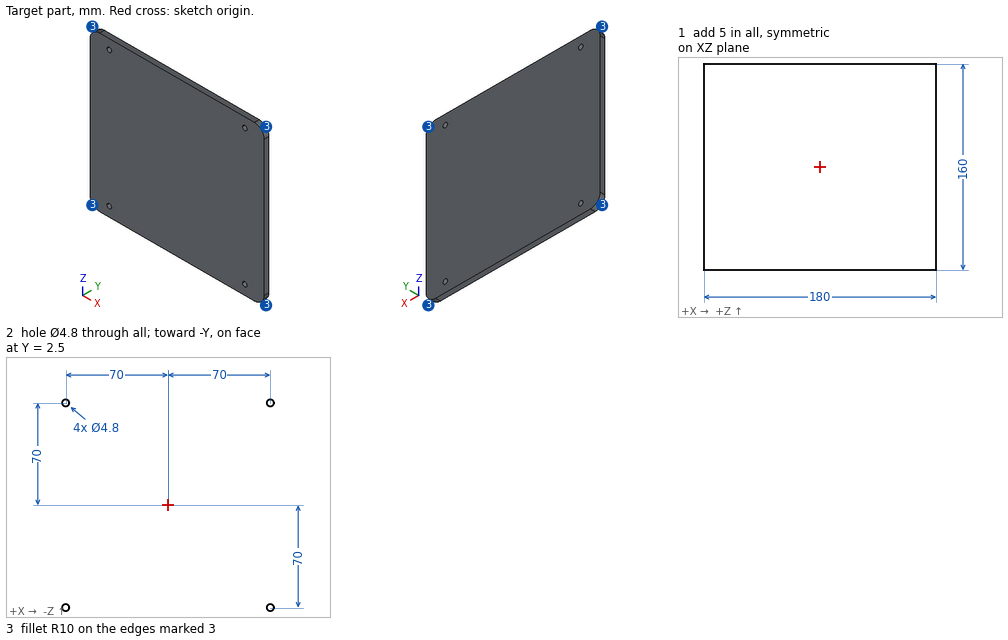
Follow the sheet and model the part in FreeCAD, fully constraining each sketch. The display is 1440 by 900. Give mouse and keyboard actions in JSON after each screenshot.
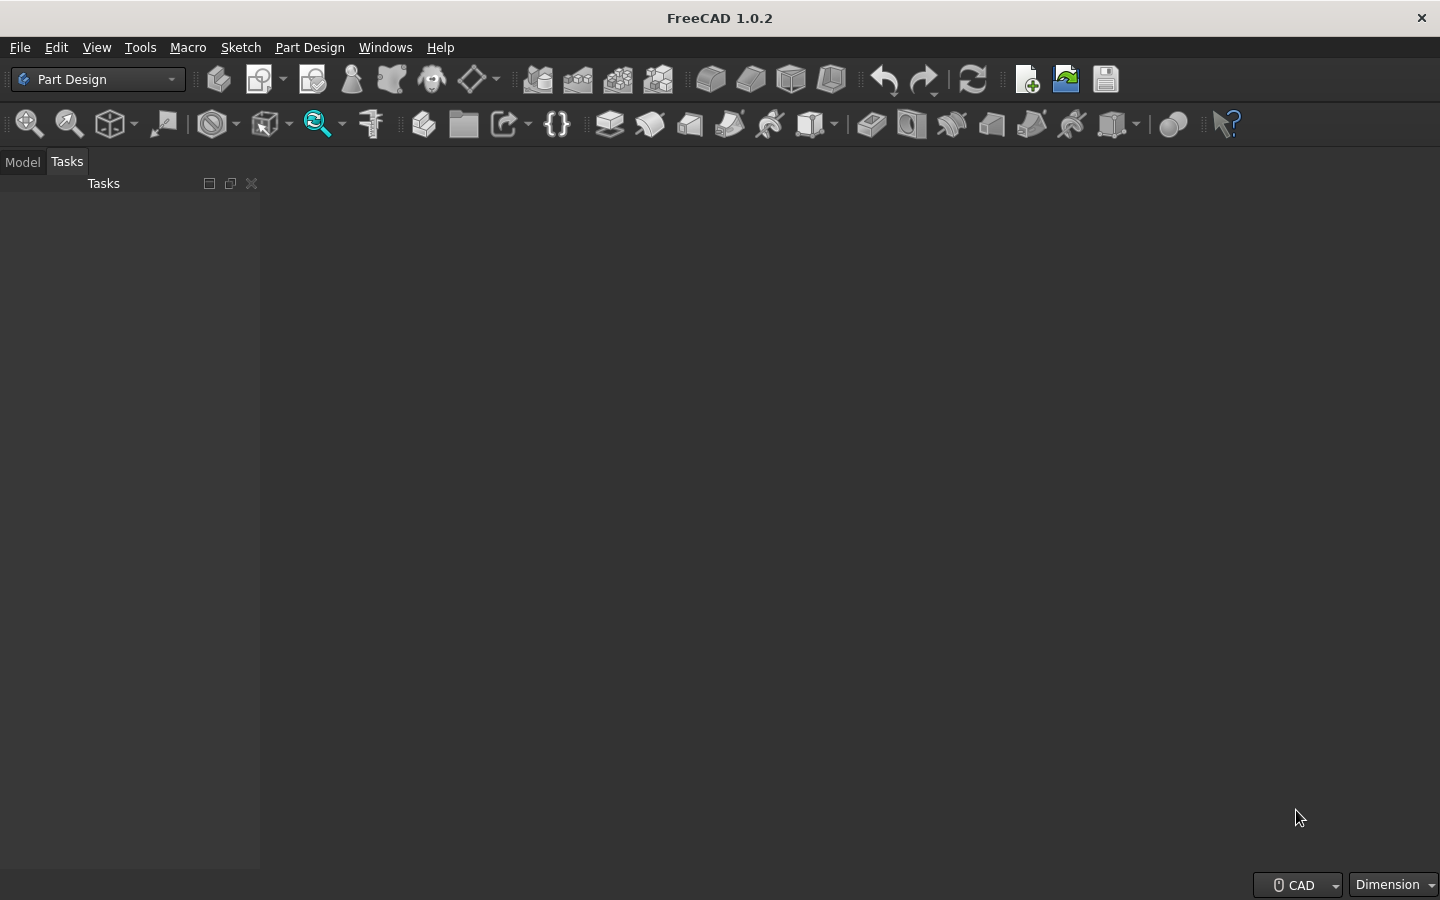
{"action": "left_click", "coordinate": [1026, 80]}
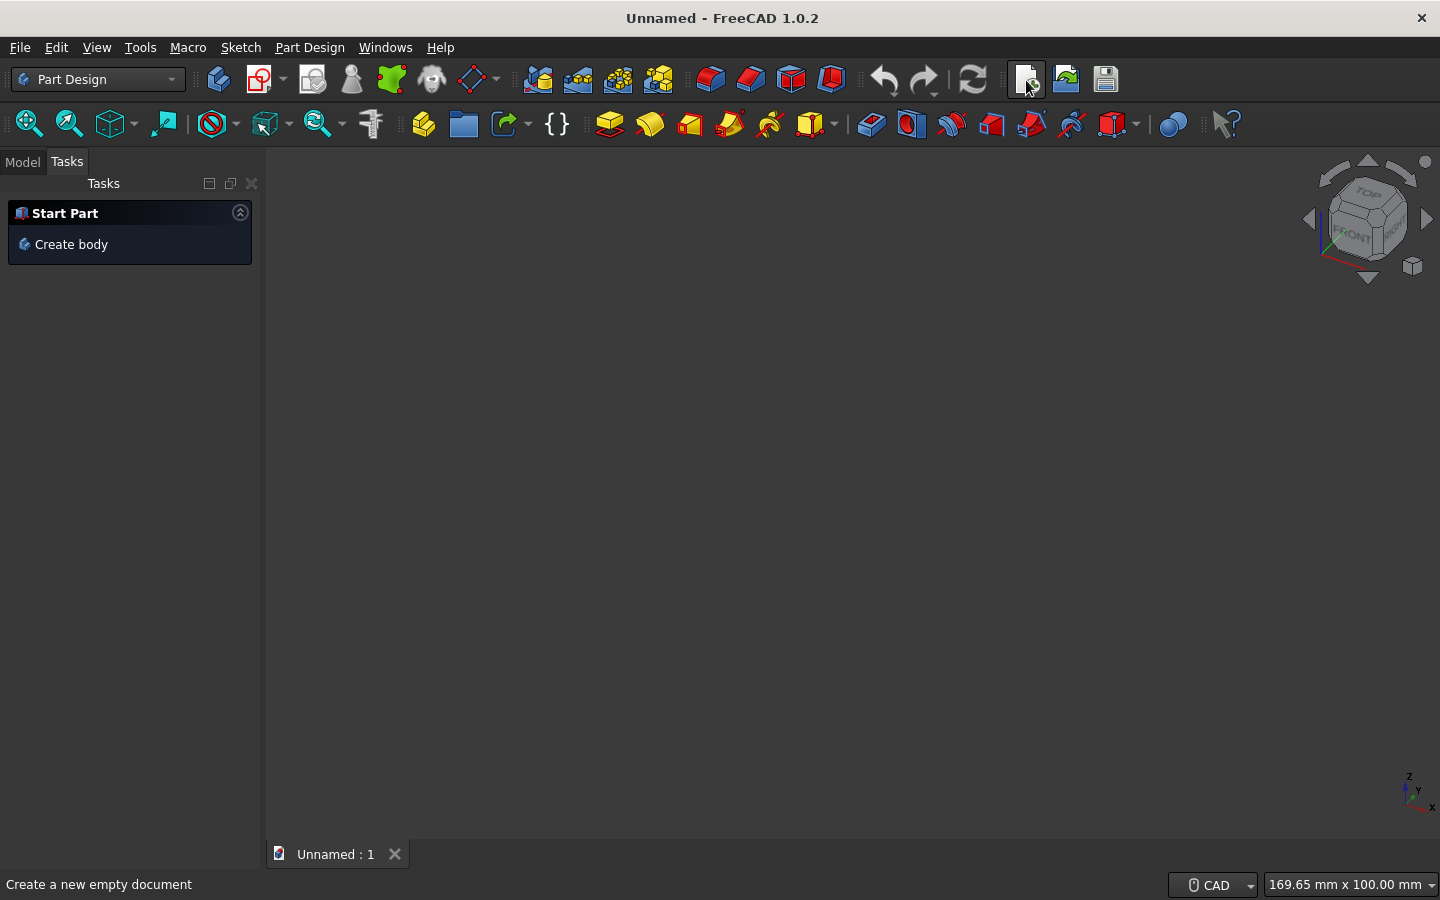
{"action": "left_click", "coordinate": [260, 80]}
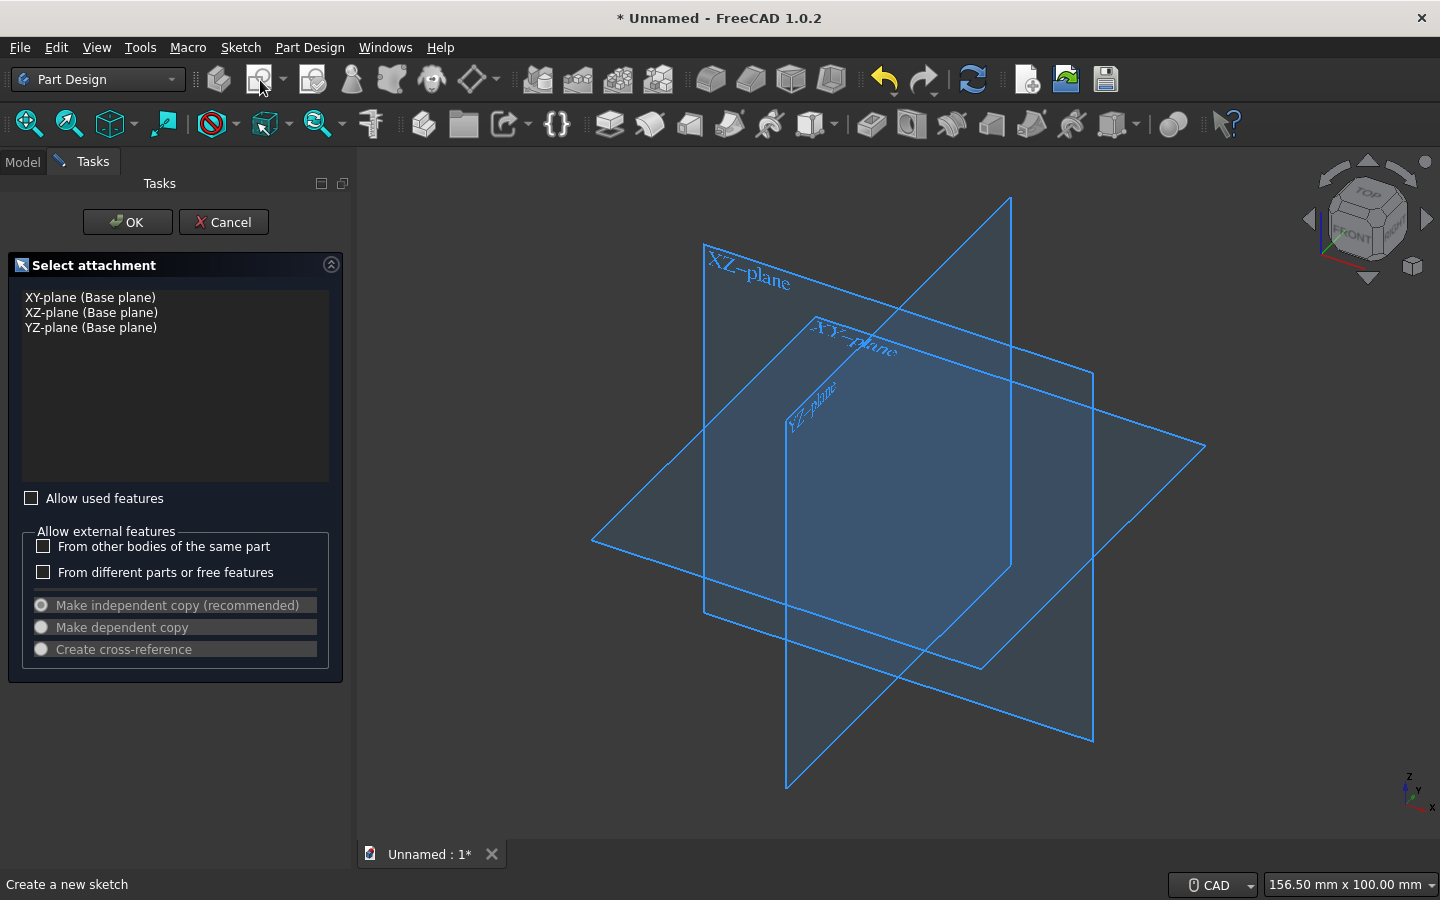
{"action": "left_click", "coordinate": [82, 312]}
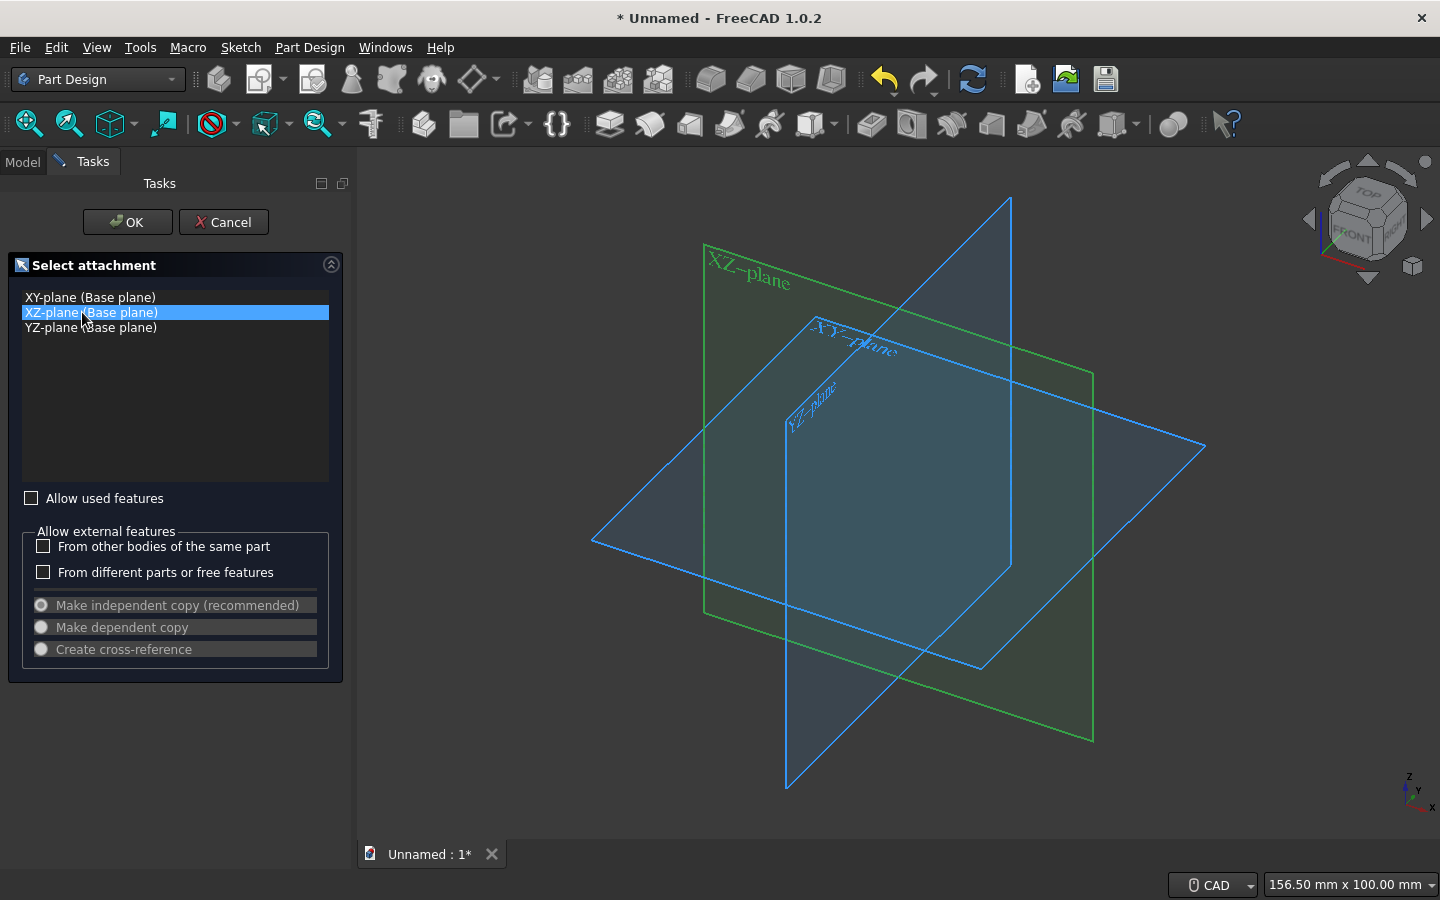
{"action": "left_click", "coordinate": [128, 222]}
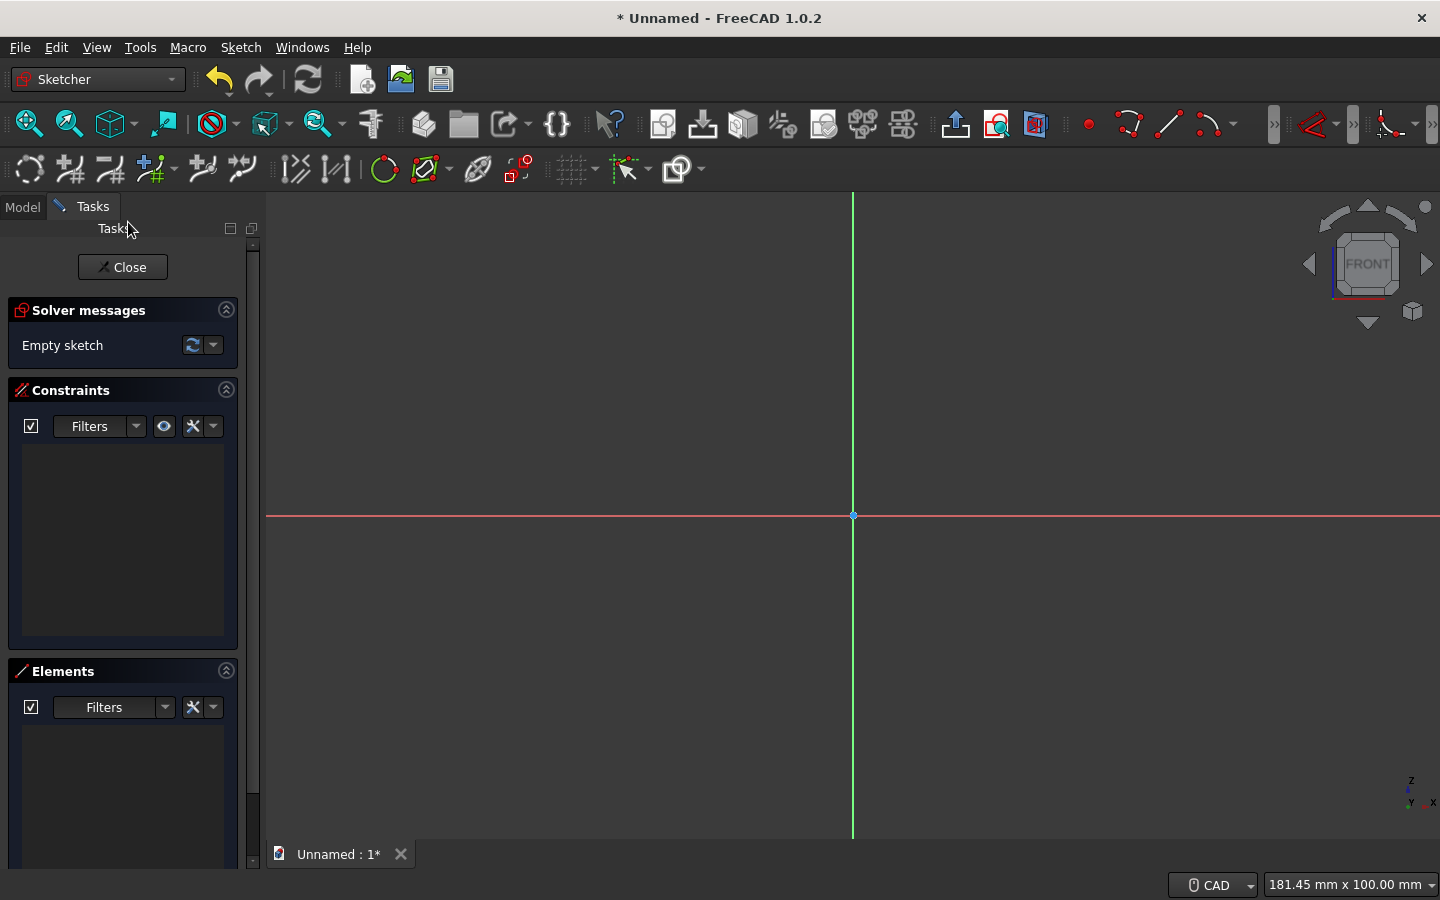
{"action": "scroll", "coordinate": [745, 515], "scroll_direction": "down", "scroll_amount": 5}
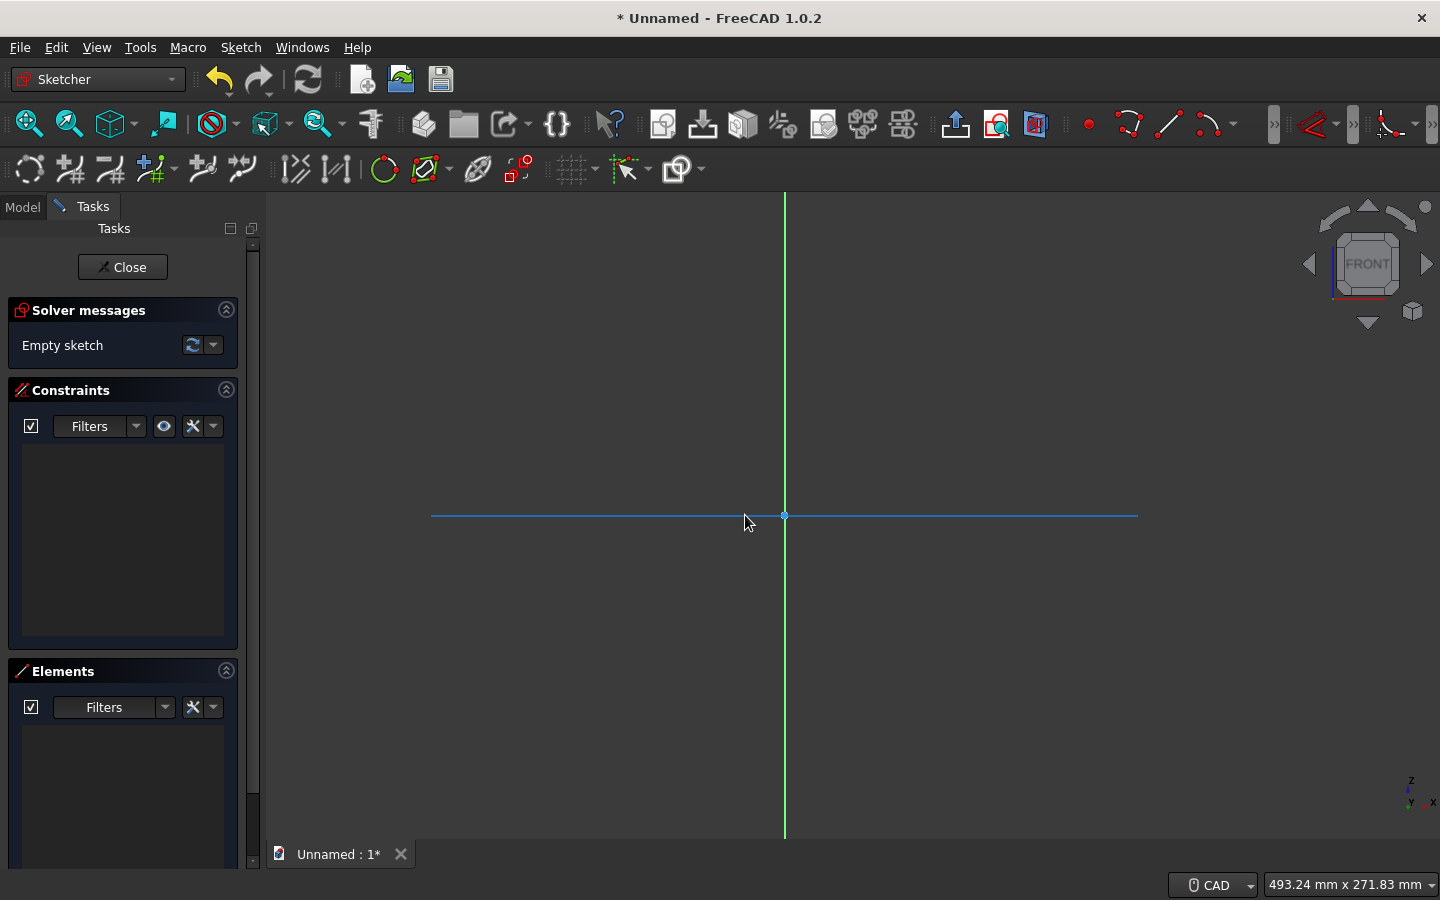
{"action": "key", "text": "g v"}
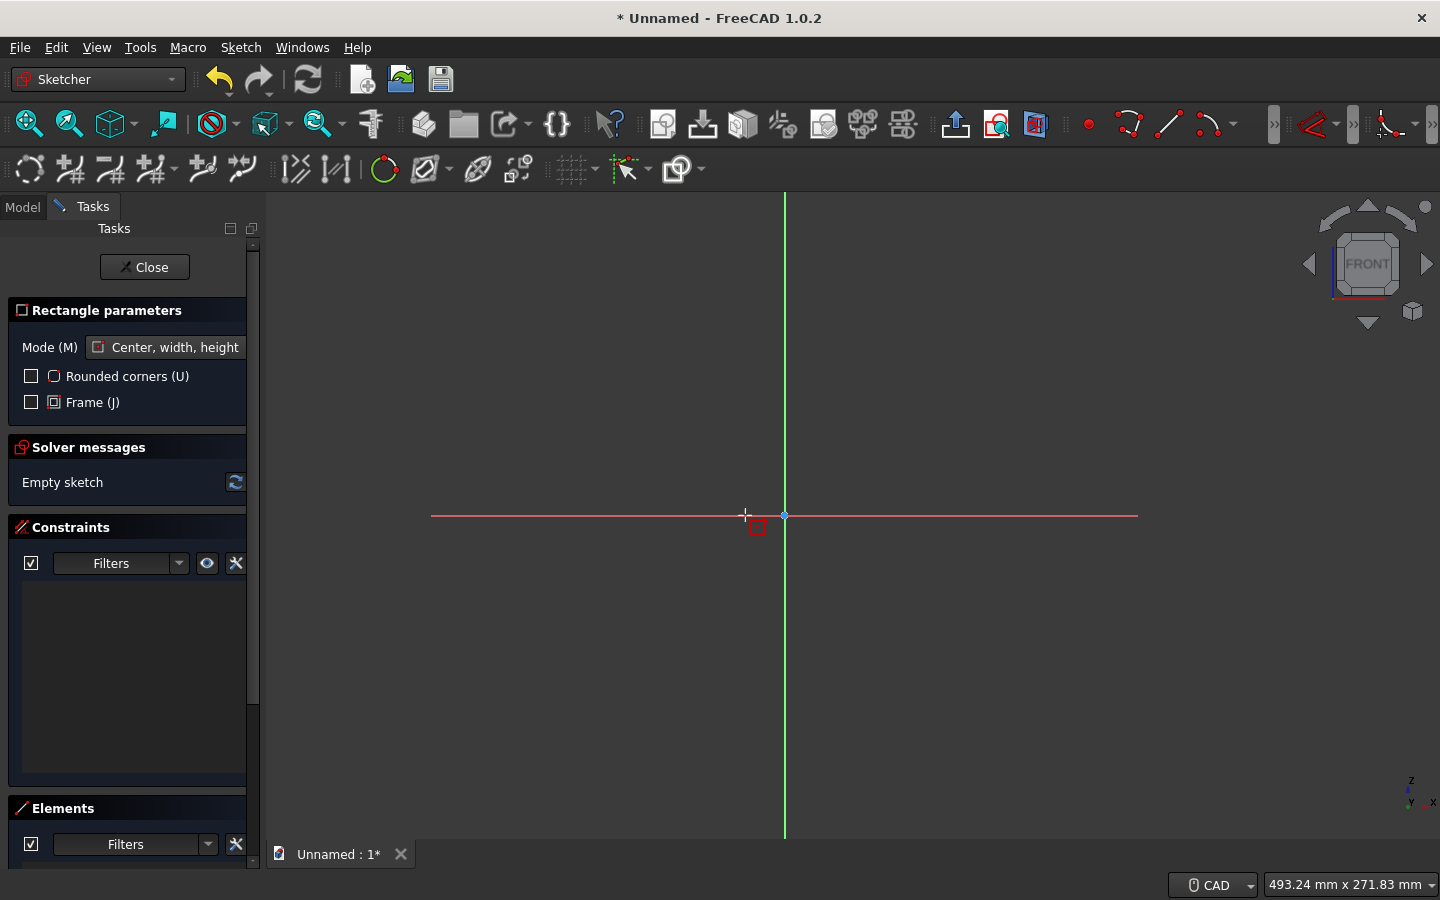
{"action": "left_click", "coordinate": [785, 516]}
{"action": "left_click", "coordinate": [999, 325]}
{"action": "key", "text": "Escape"}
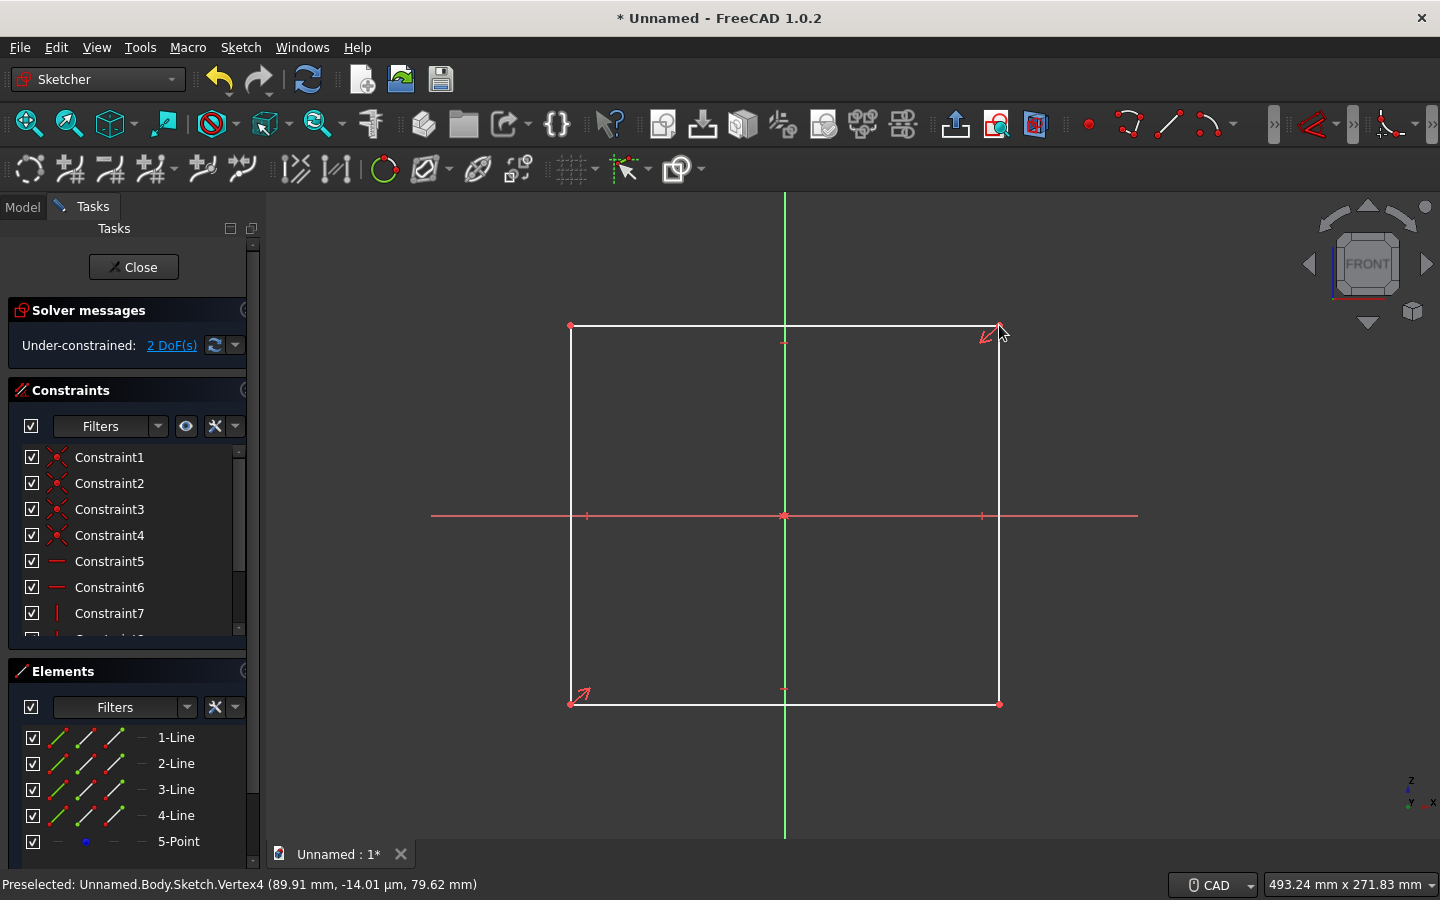
{"action": "left_click", "coordinate": [1312, 124]}